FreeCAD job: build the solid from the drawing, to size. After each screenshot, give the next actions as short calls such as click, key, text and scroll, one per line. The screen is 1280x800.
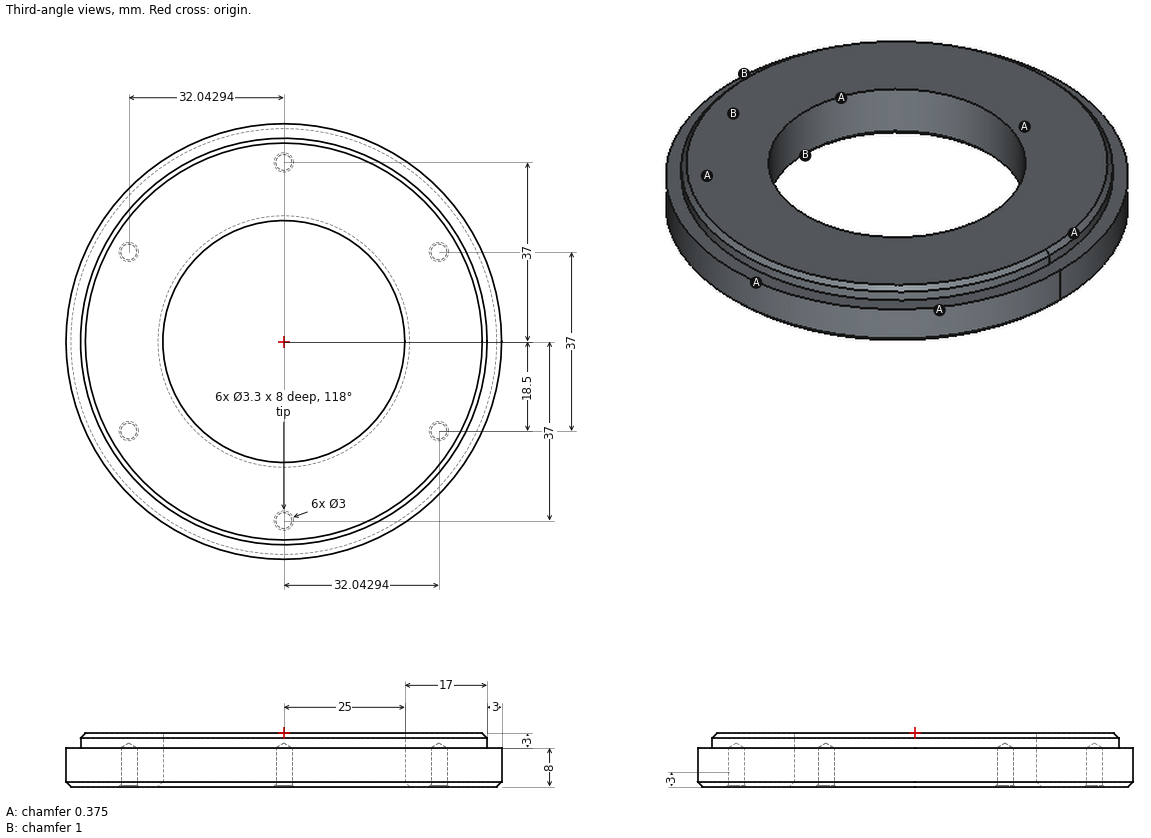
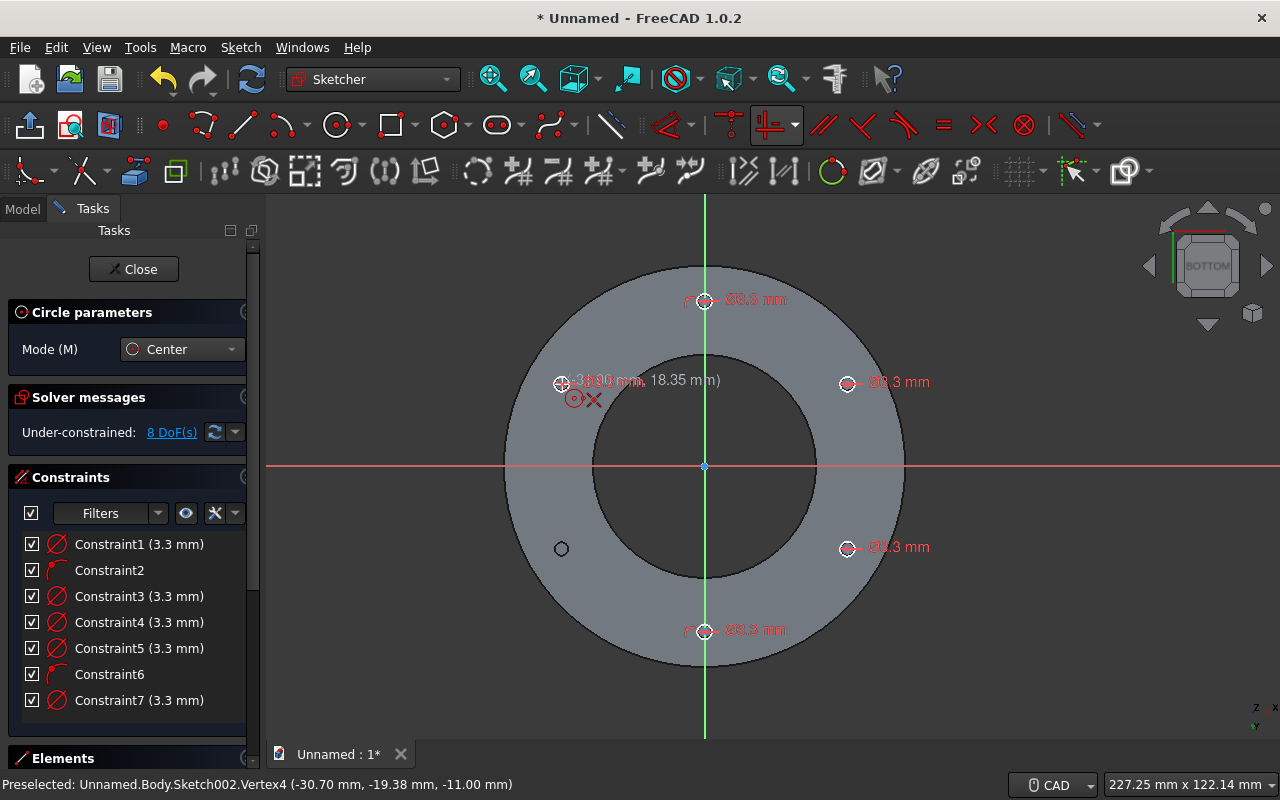
scroll(562, 549, up, 6)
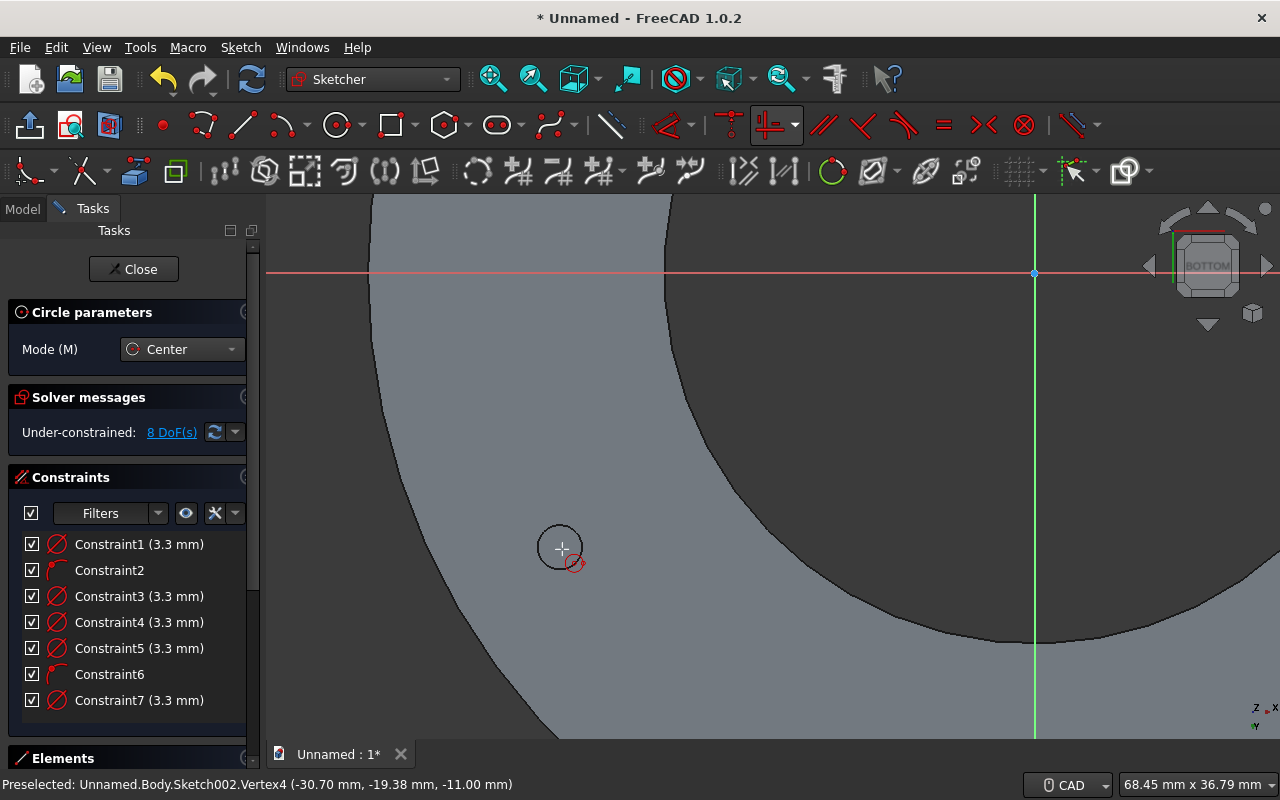
click(560, 547)
move(577, 530)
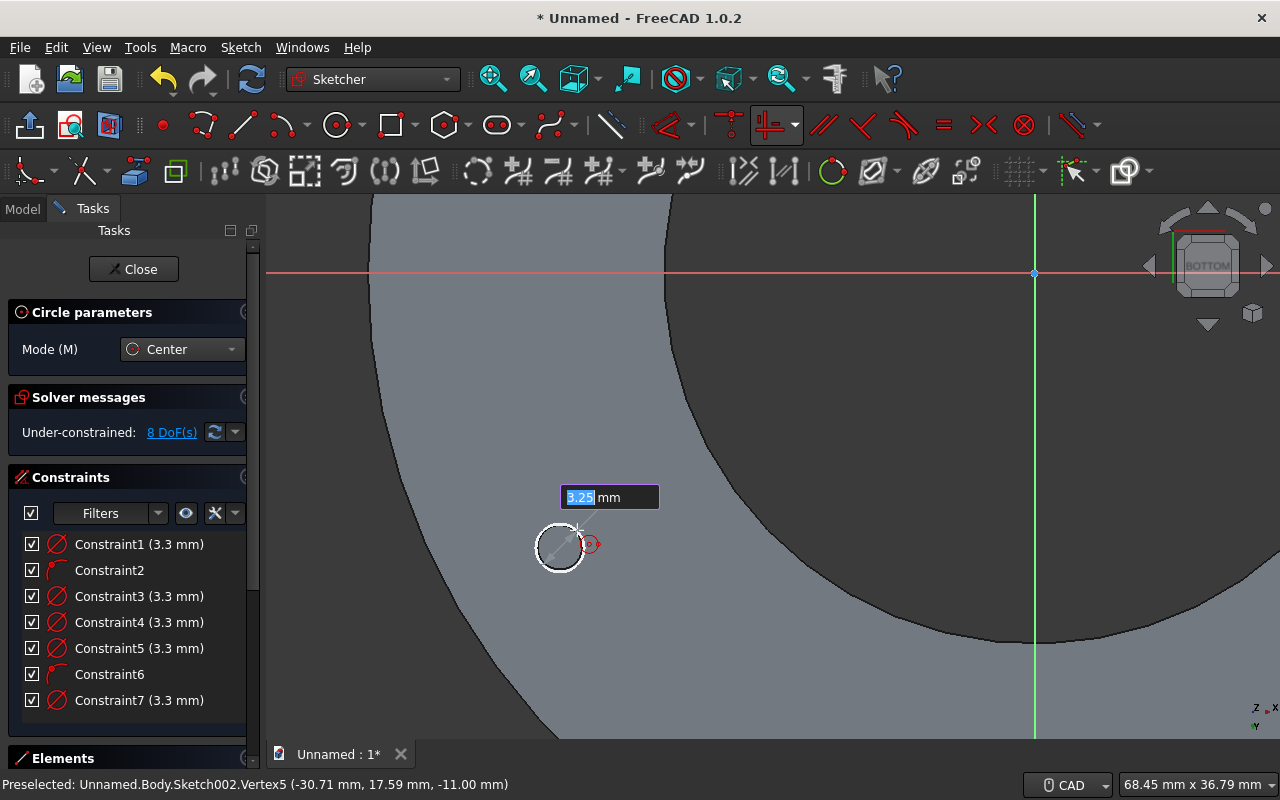
text(3.3)
key(Return)
key(Escape)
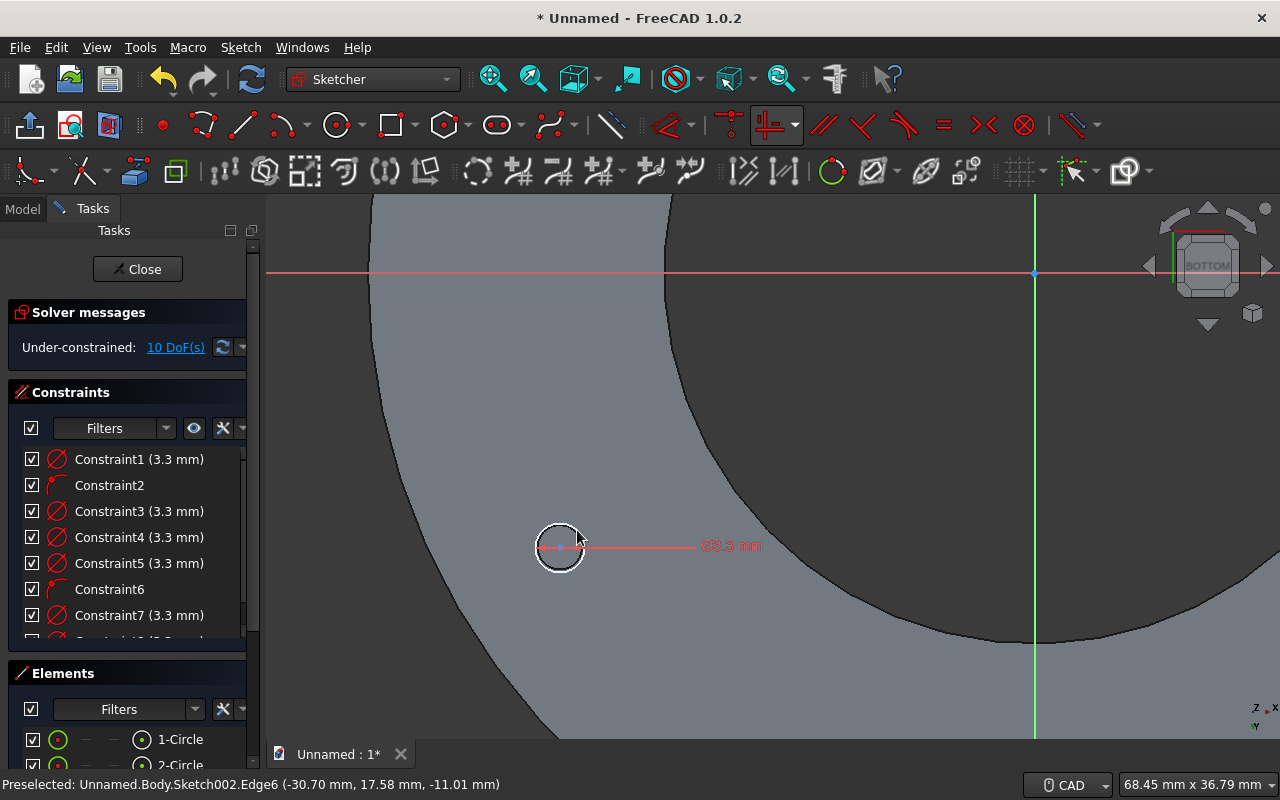
scroll(562, 550, down, 6)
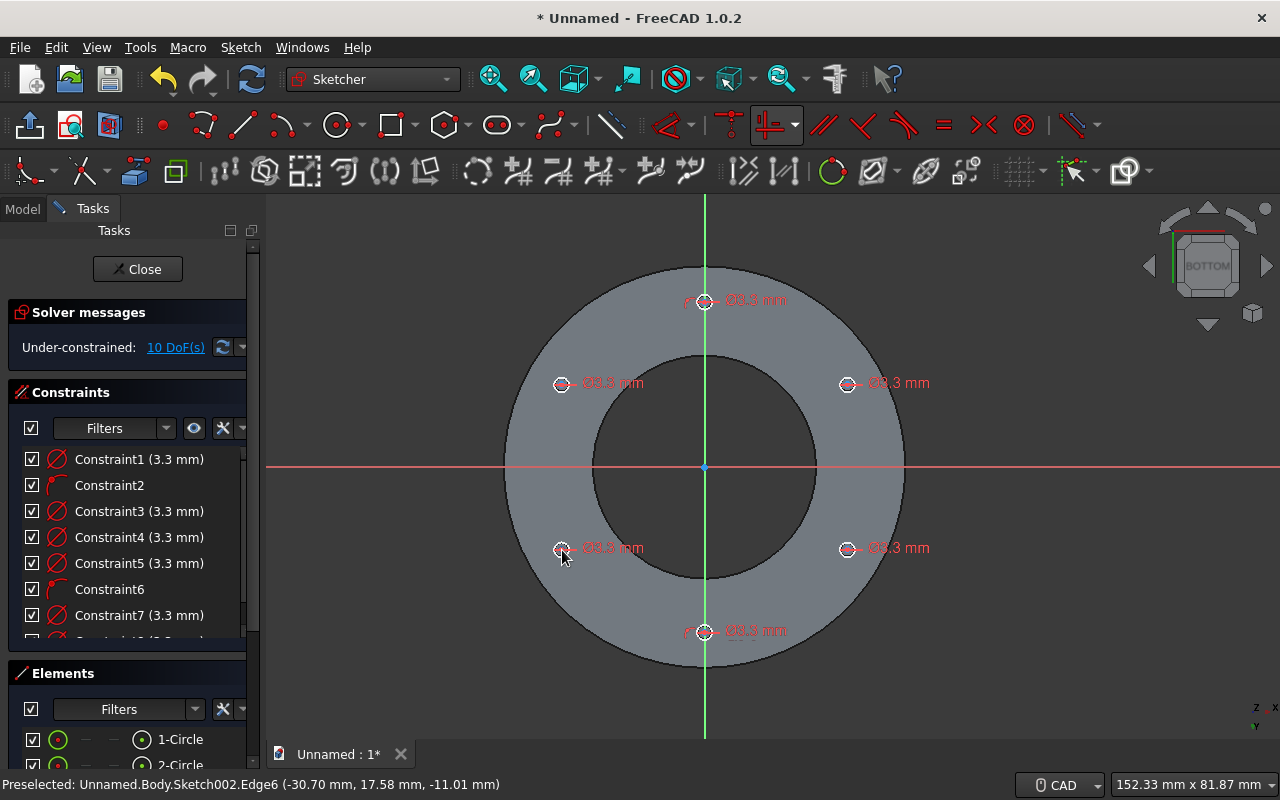
click(847, 385)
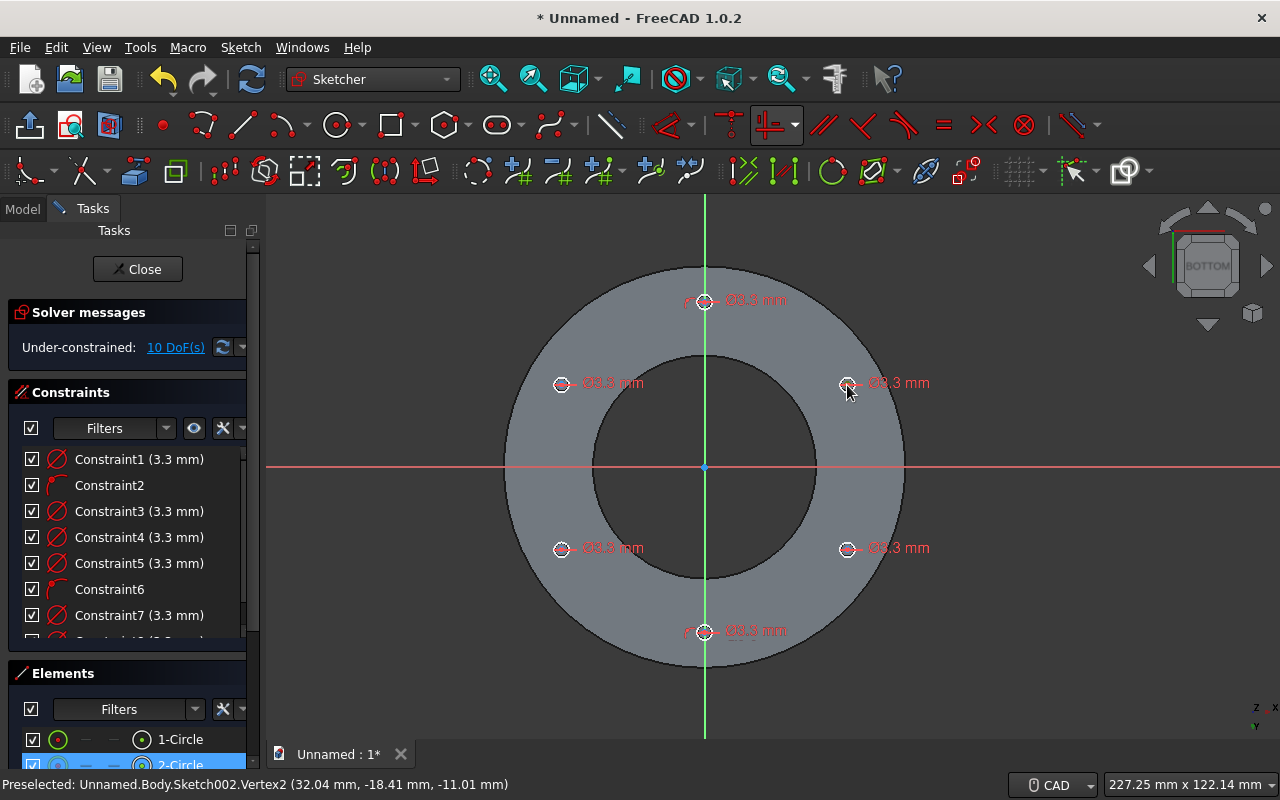
click(847, 550)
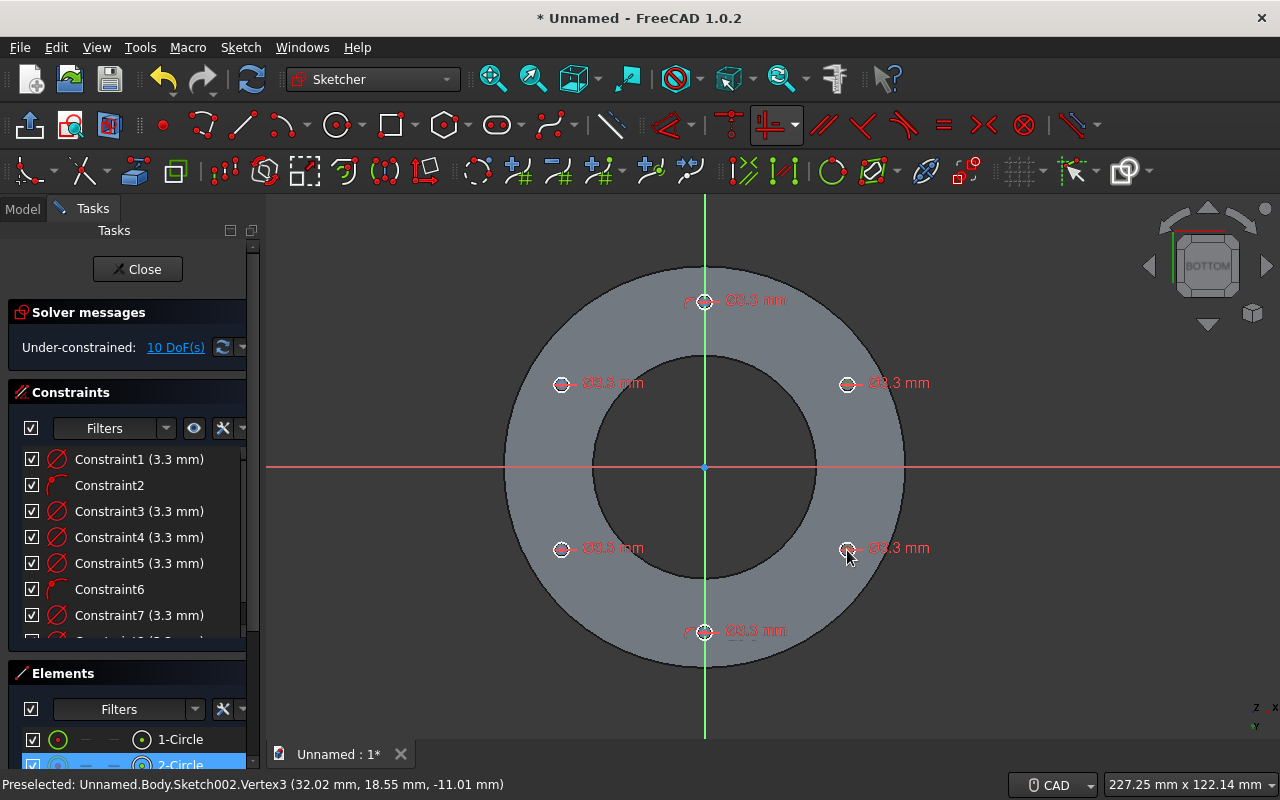
click(798, 126)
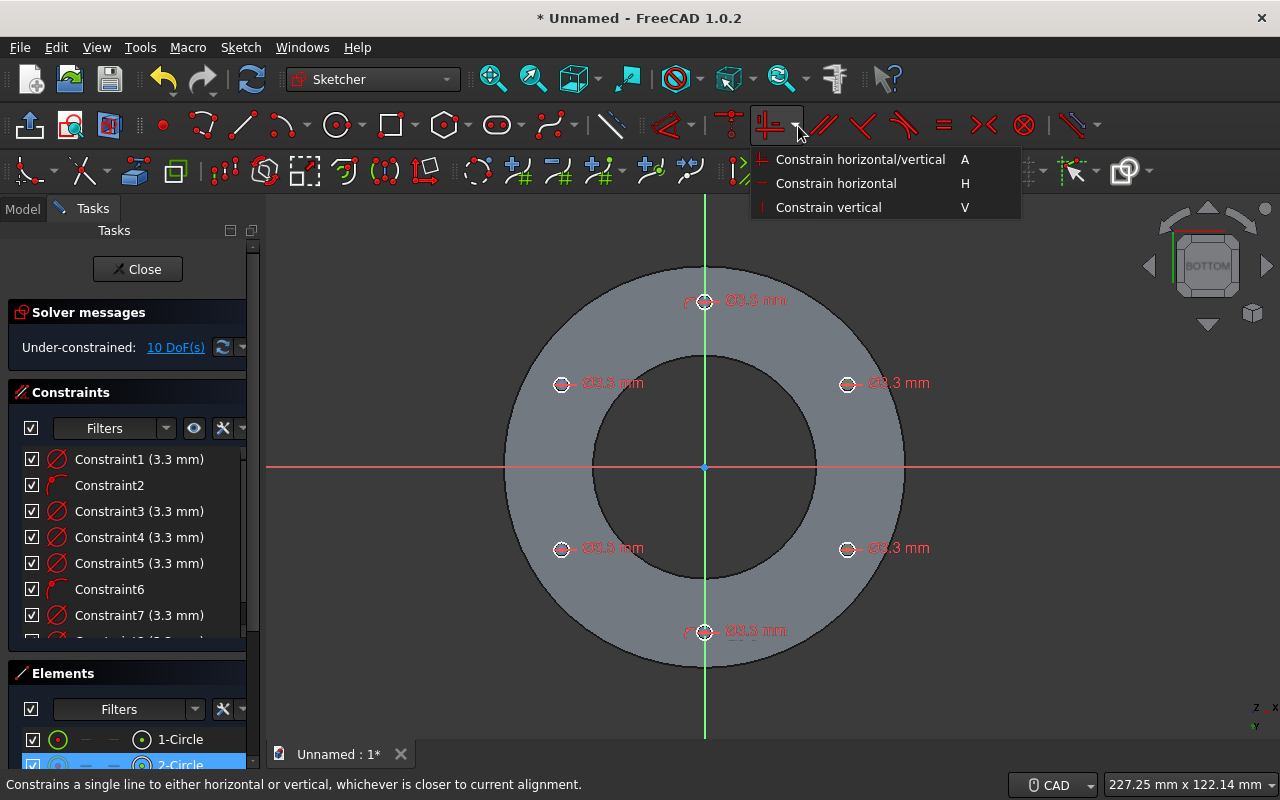
click(886, 207)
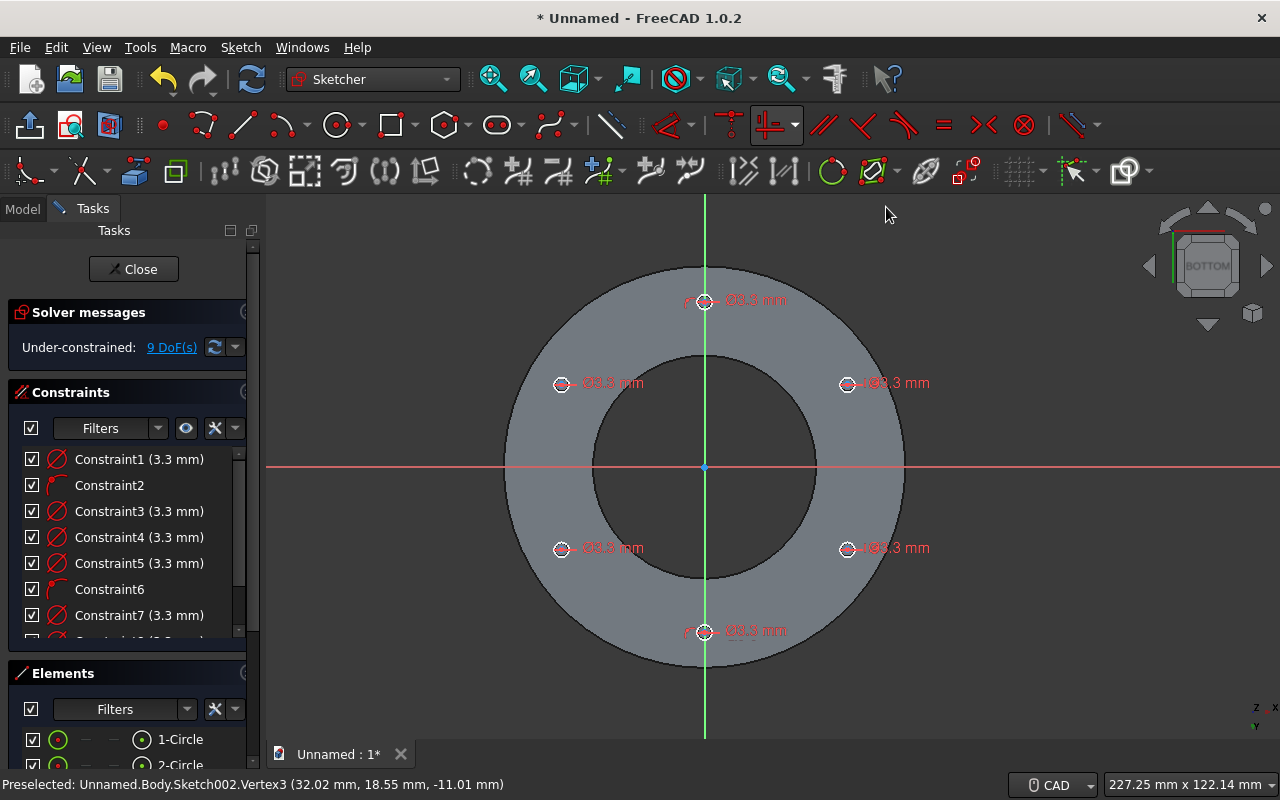
click(847, 385)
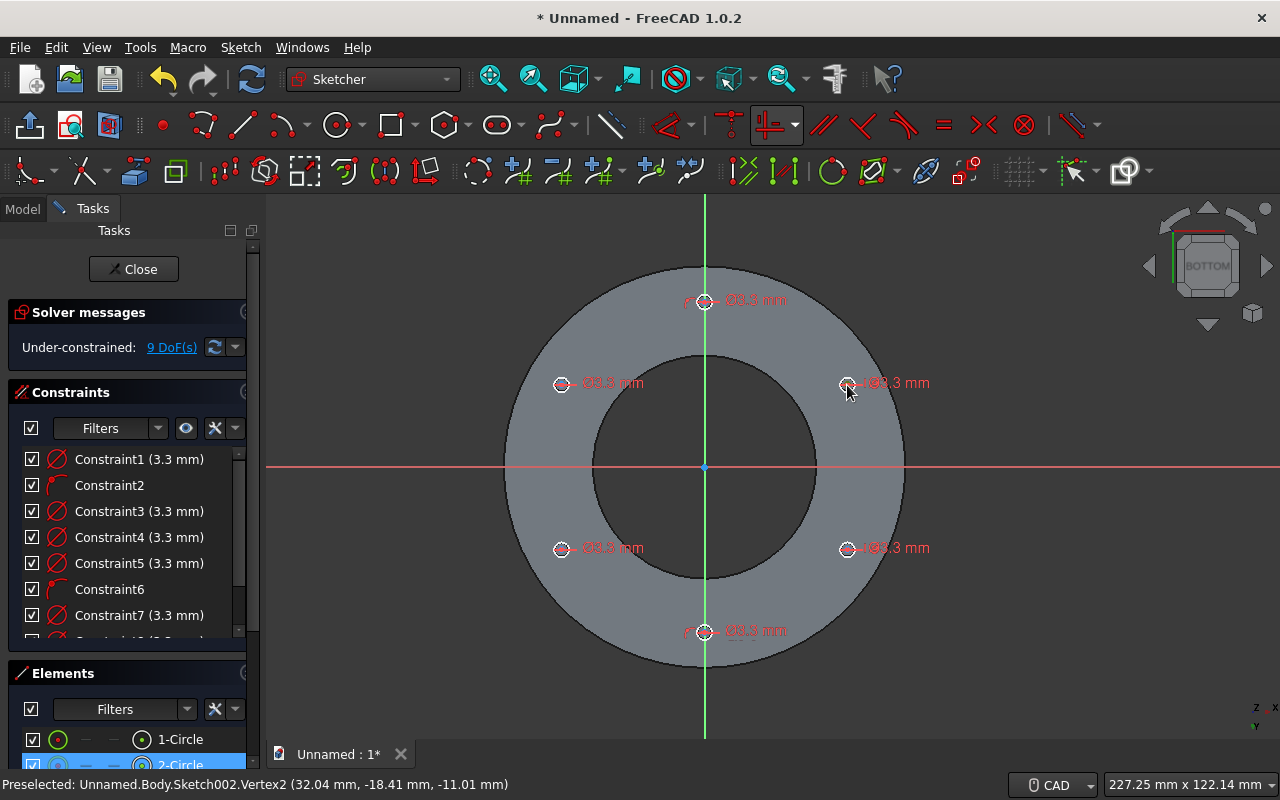
click(562, 385)